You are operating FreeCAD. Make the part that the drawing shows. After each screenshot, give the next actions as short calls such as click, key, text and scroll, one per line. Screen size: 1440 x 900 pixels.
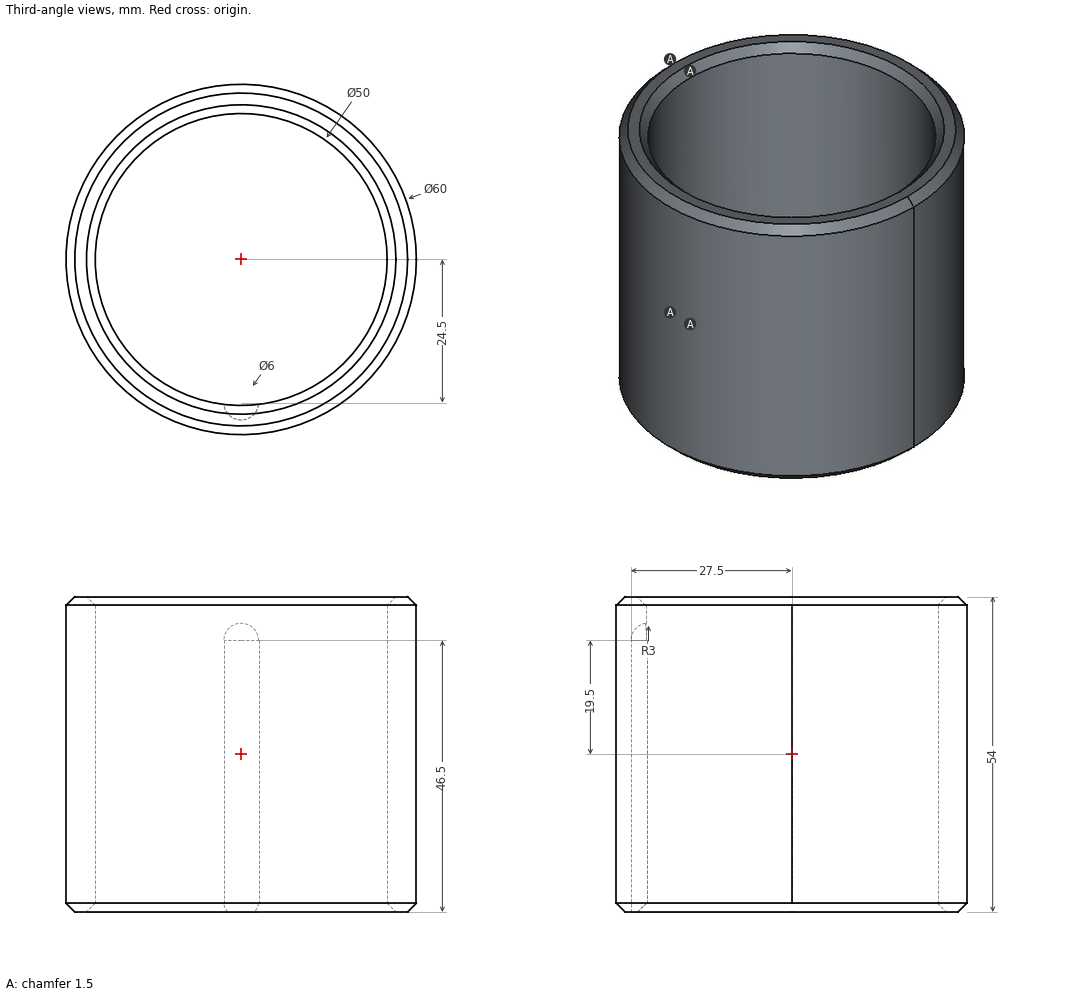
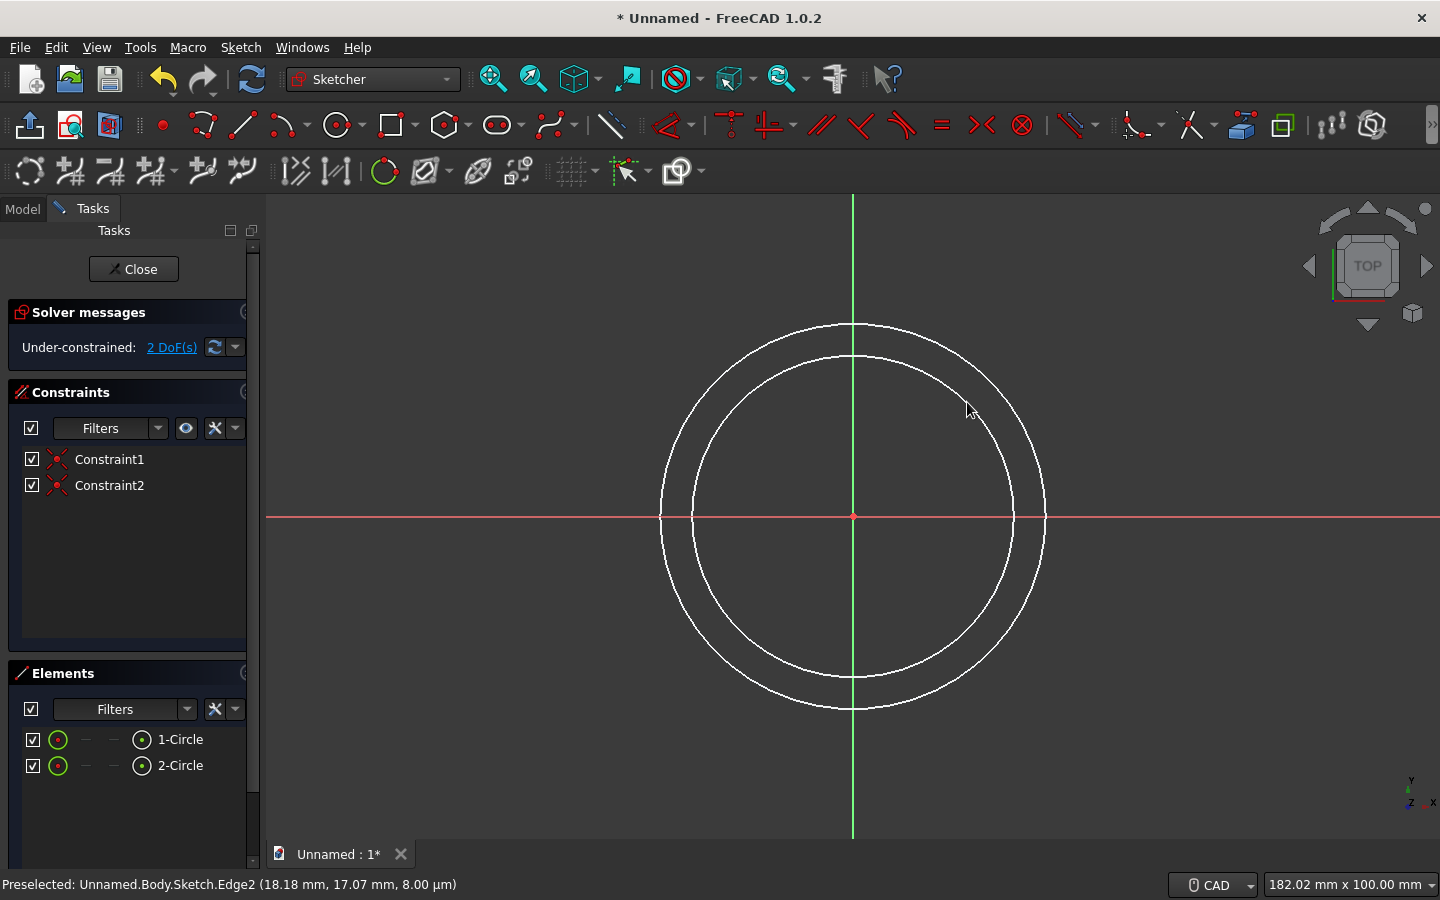
click(989, 380)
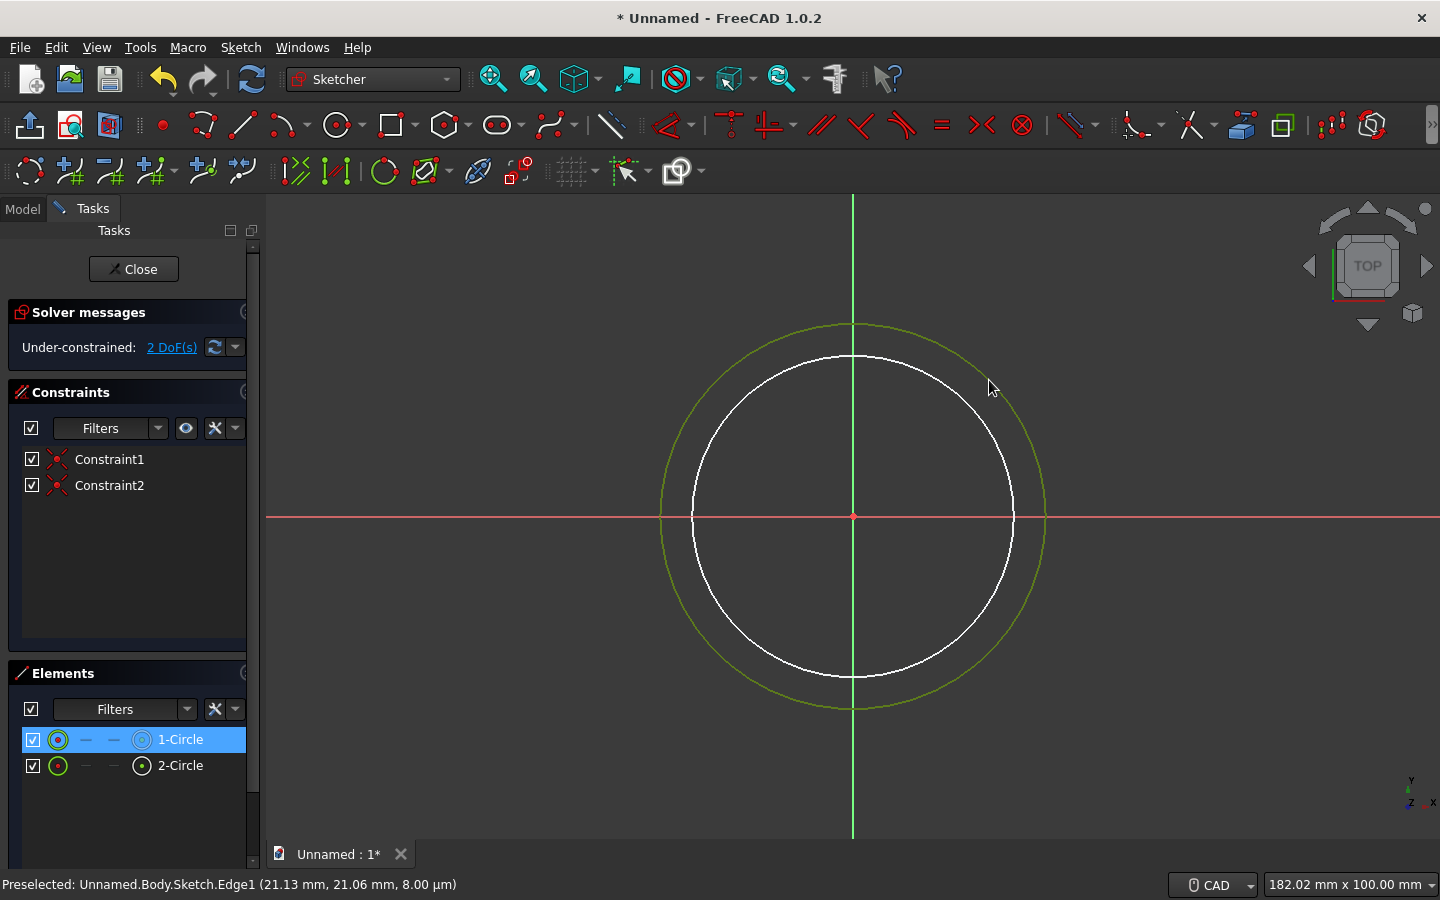
key(k)
key(o)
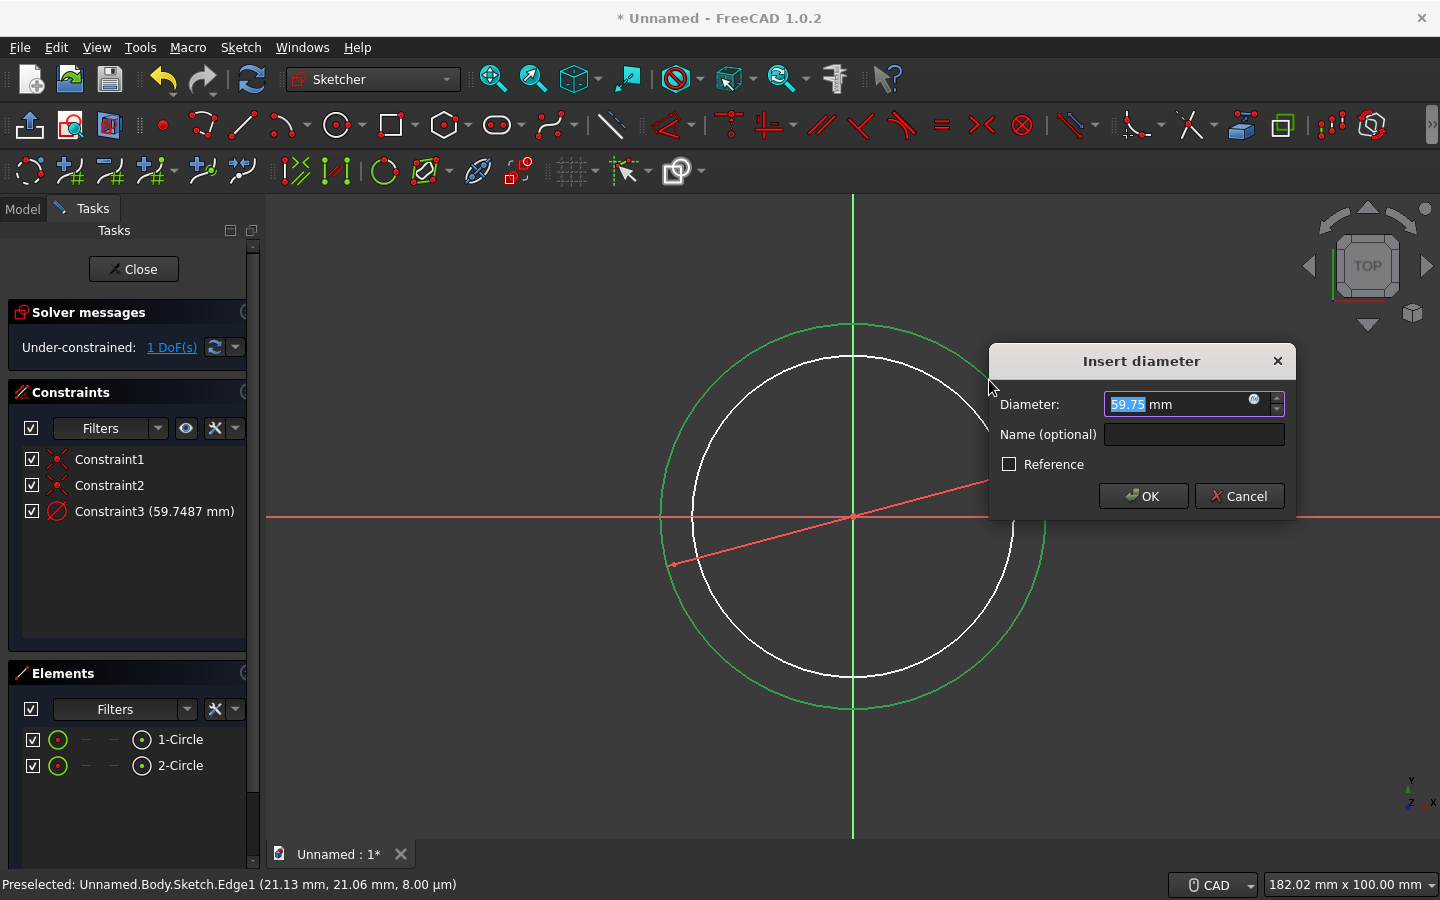
text(60)
key(Return)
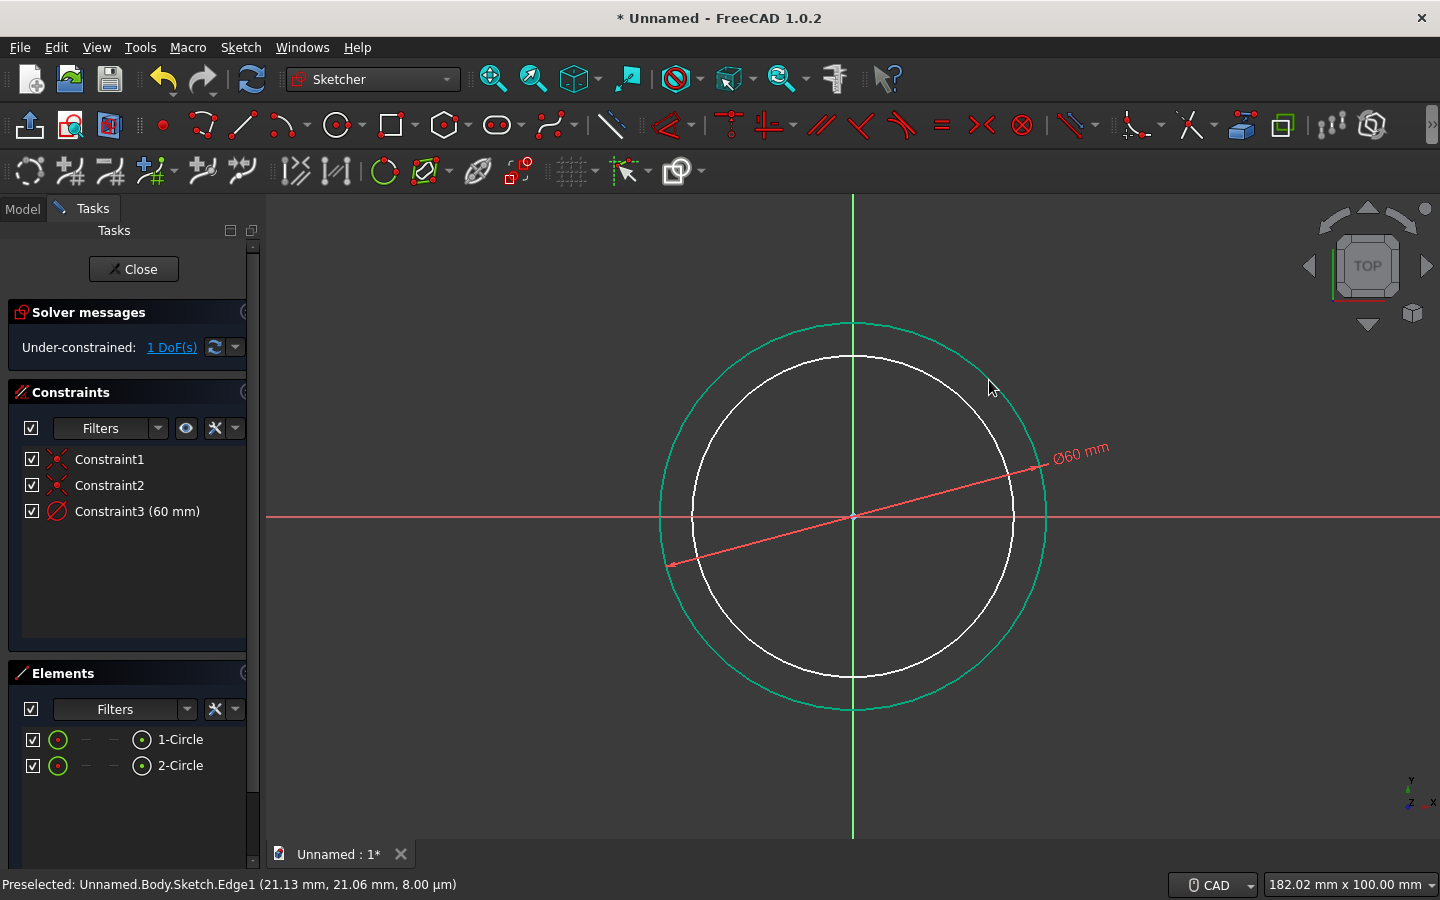
click(966, 402)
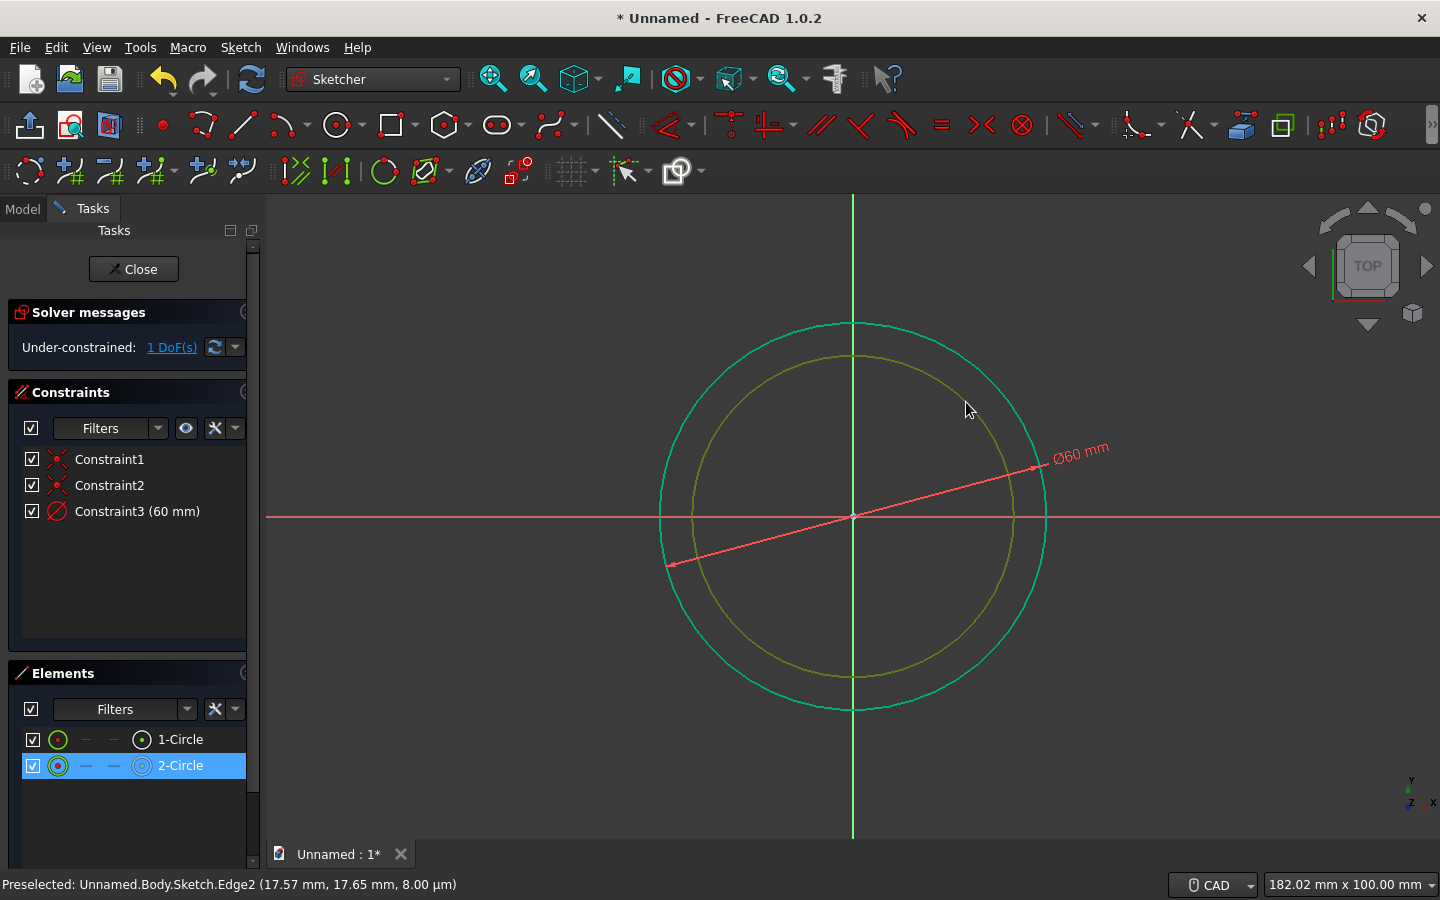
click(694, 126)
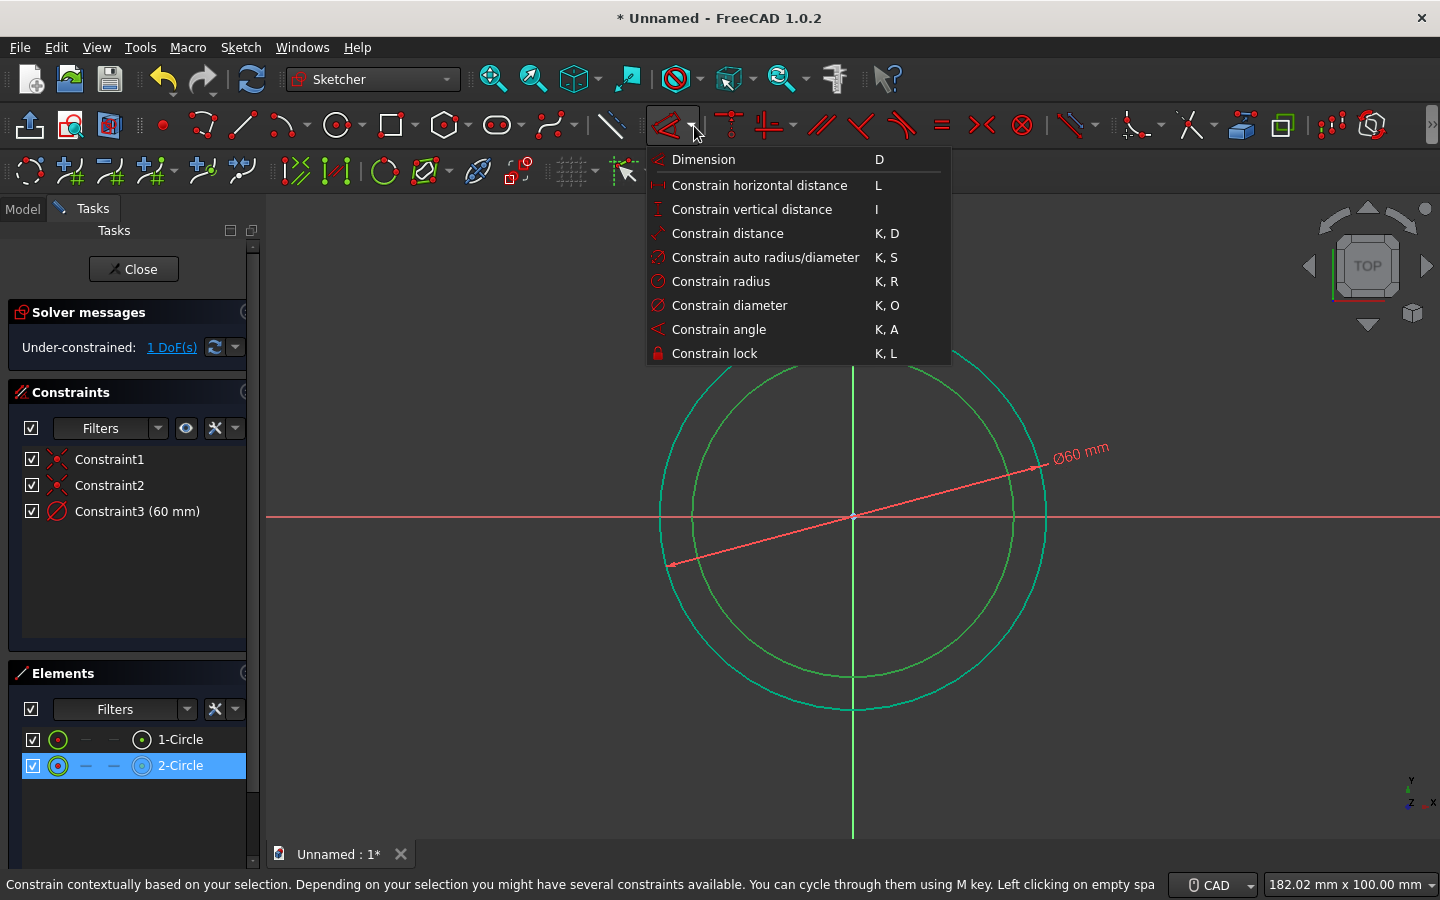
click(799, 305)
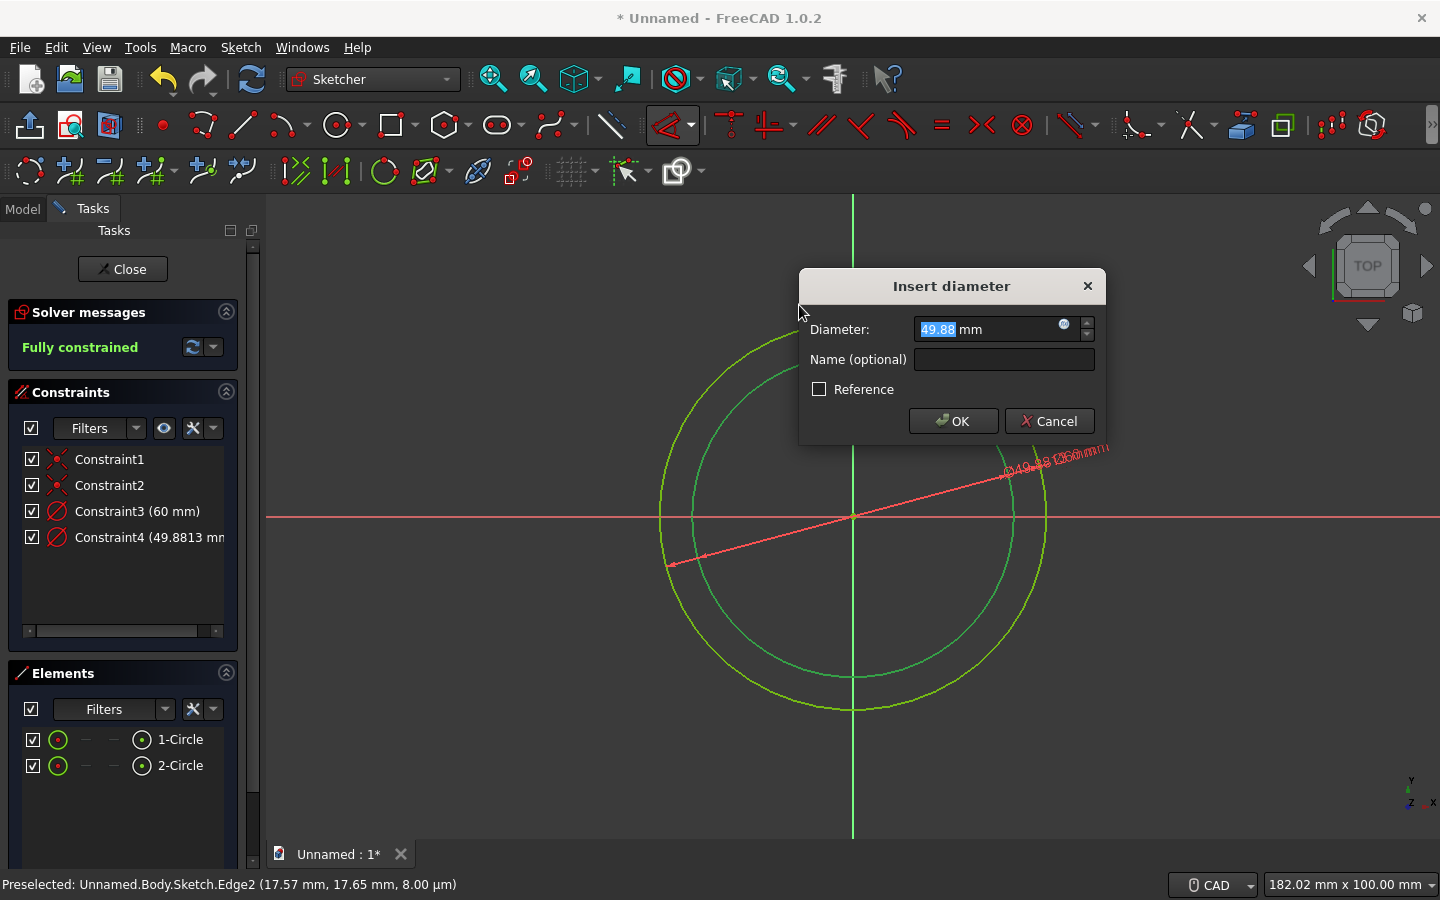
text(50)
key(Return)